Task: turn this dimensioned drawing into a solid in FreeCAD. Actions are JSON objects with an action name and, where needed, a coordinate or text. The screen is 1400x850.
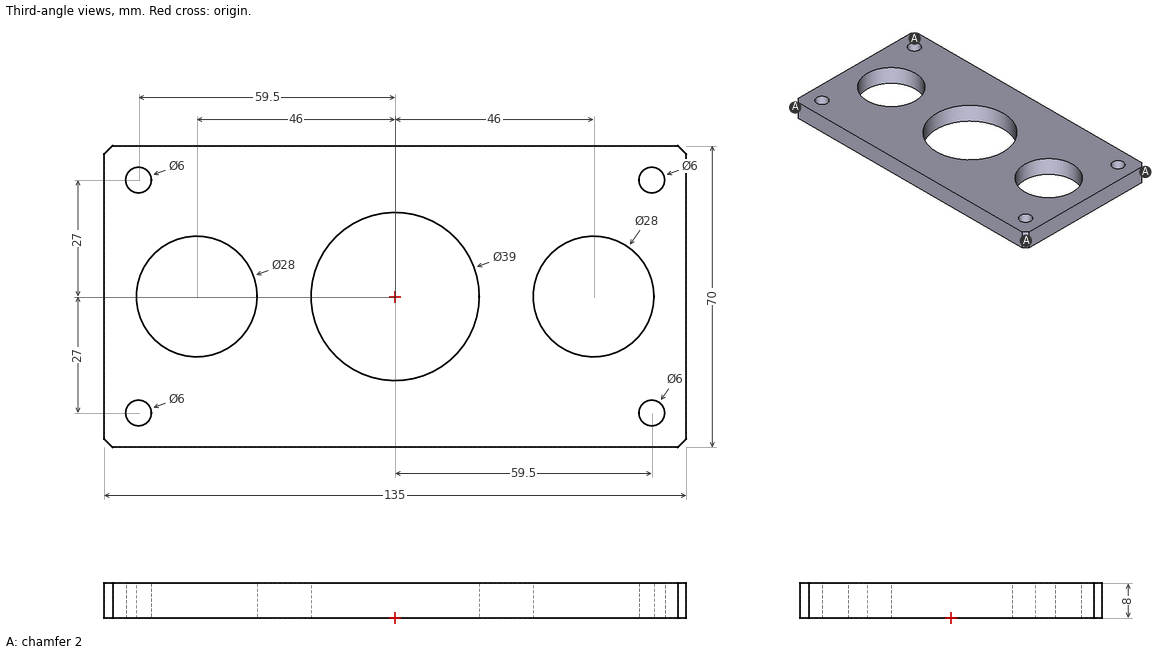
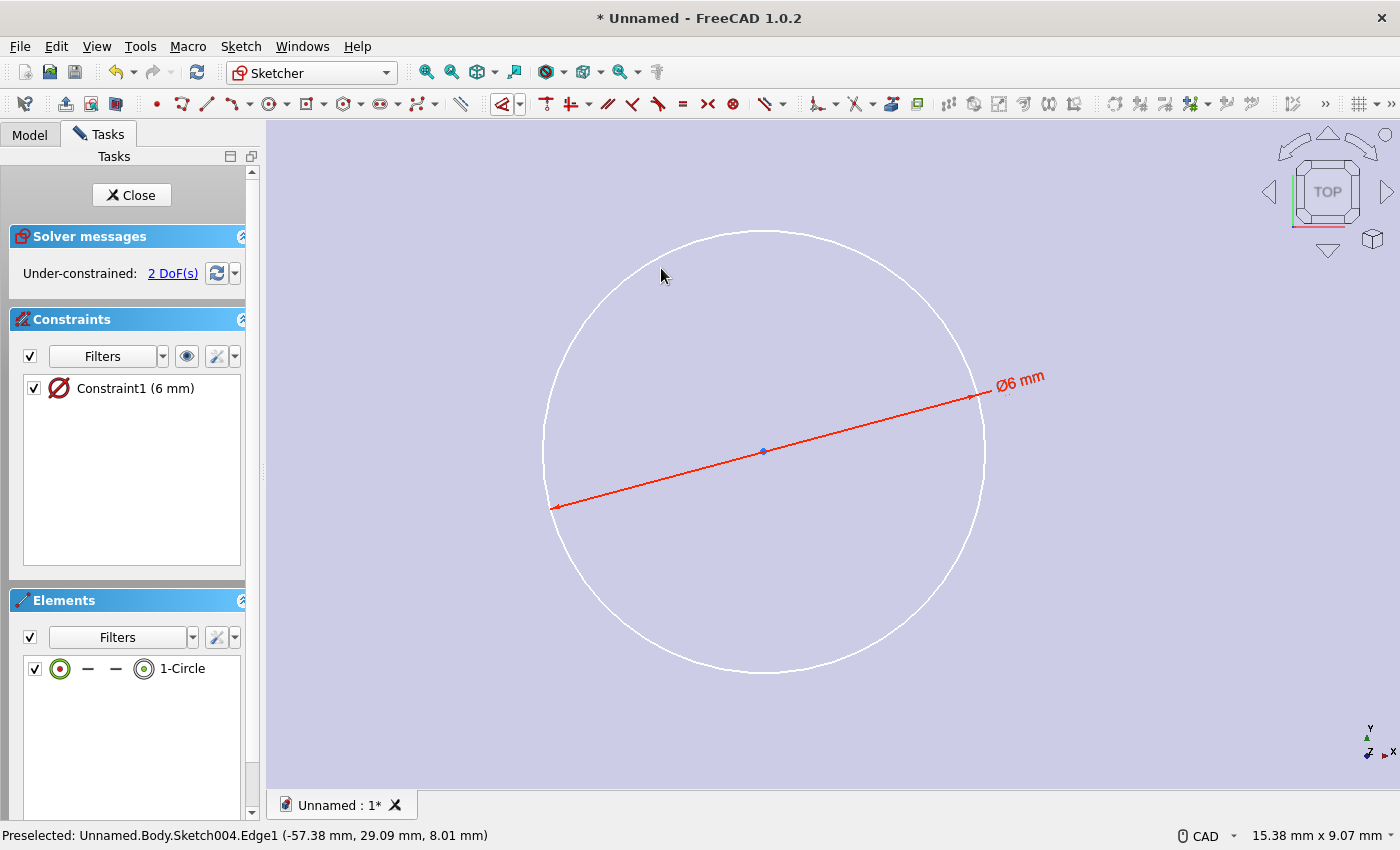
{"action": "left_click", "coordinate": [764, 452]}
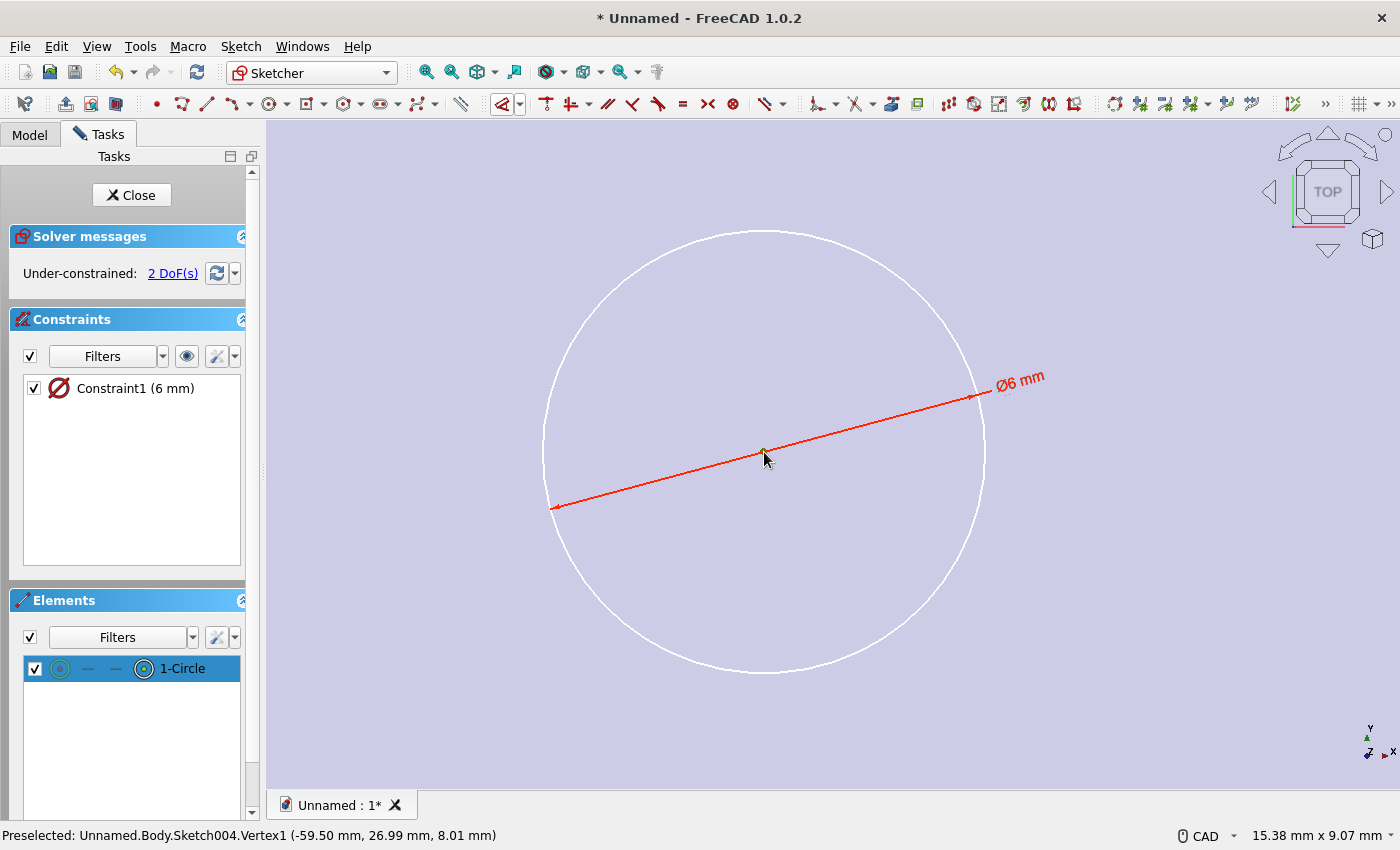
{"action": "key", "text": "i"}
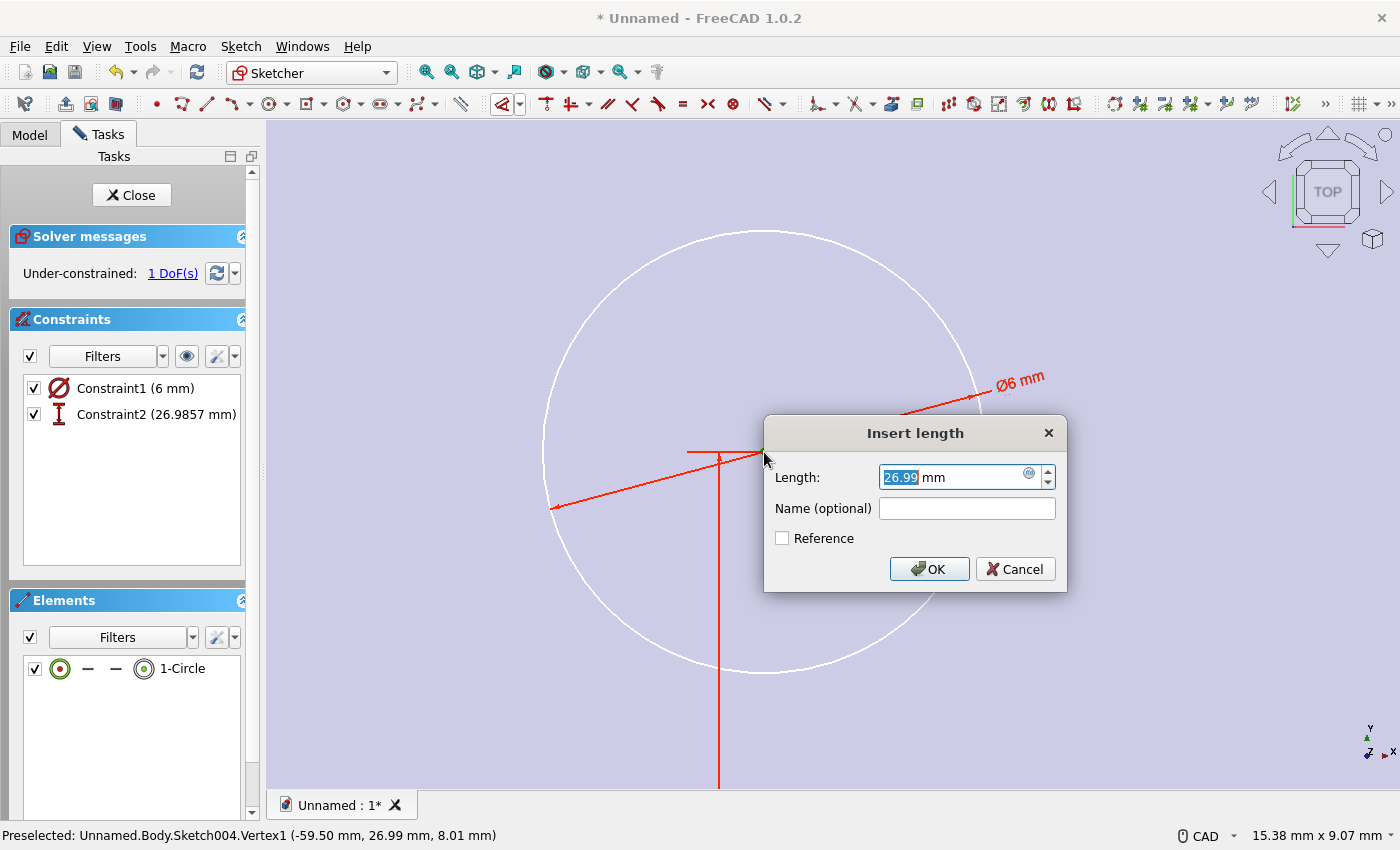
{"action": "type", "text": "27"}
{"action": "key", "text": "Return"}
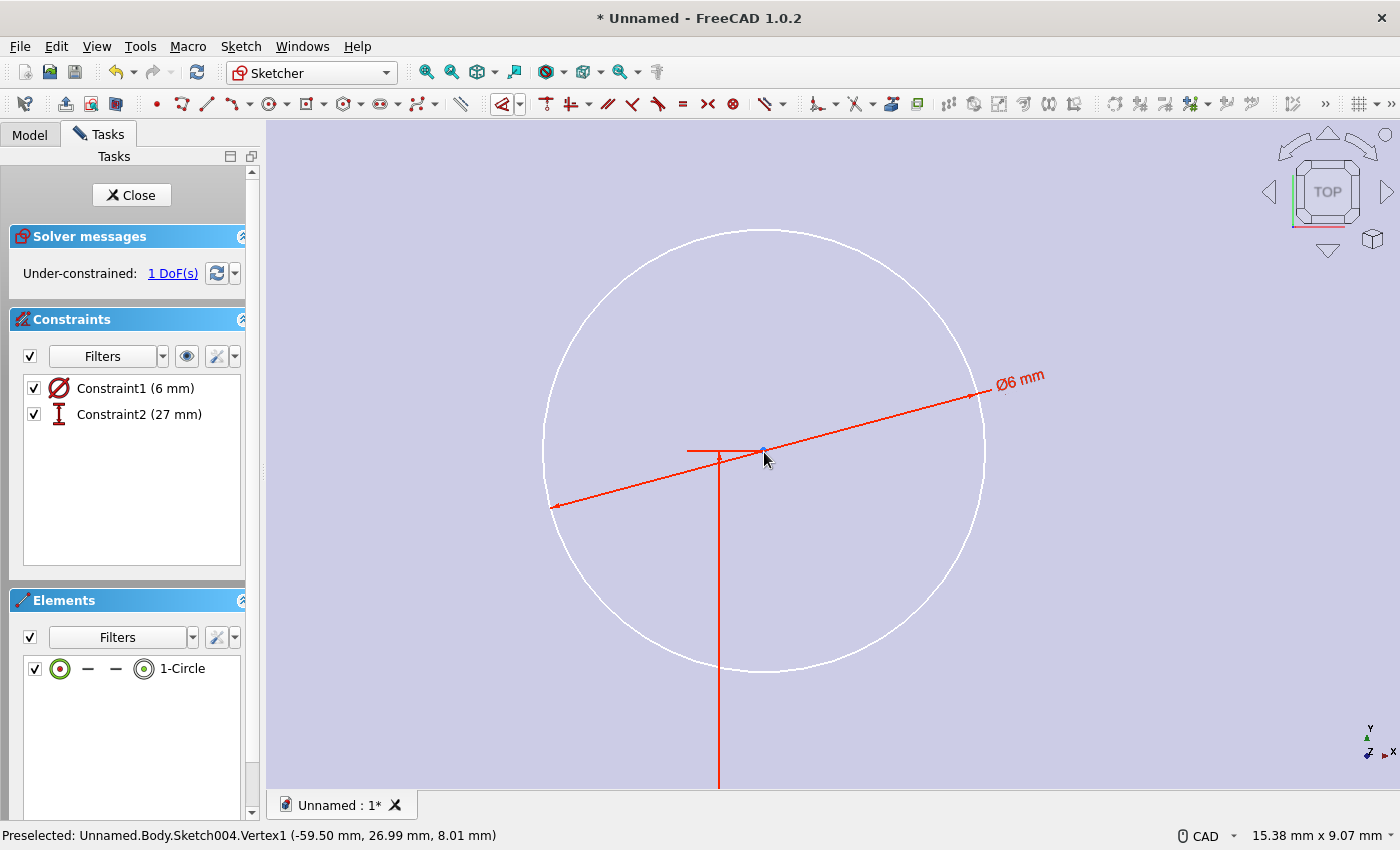
{"action": "left_click", "coordinate": [764, 451]}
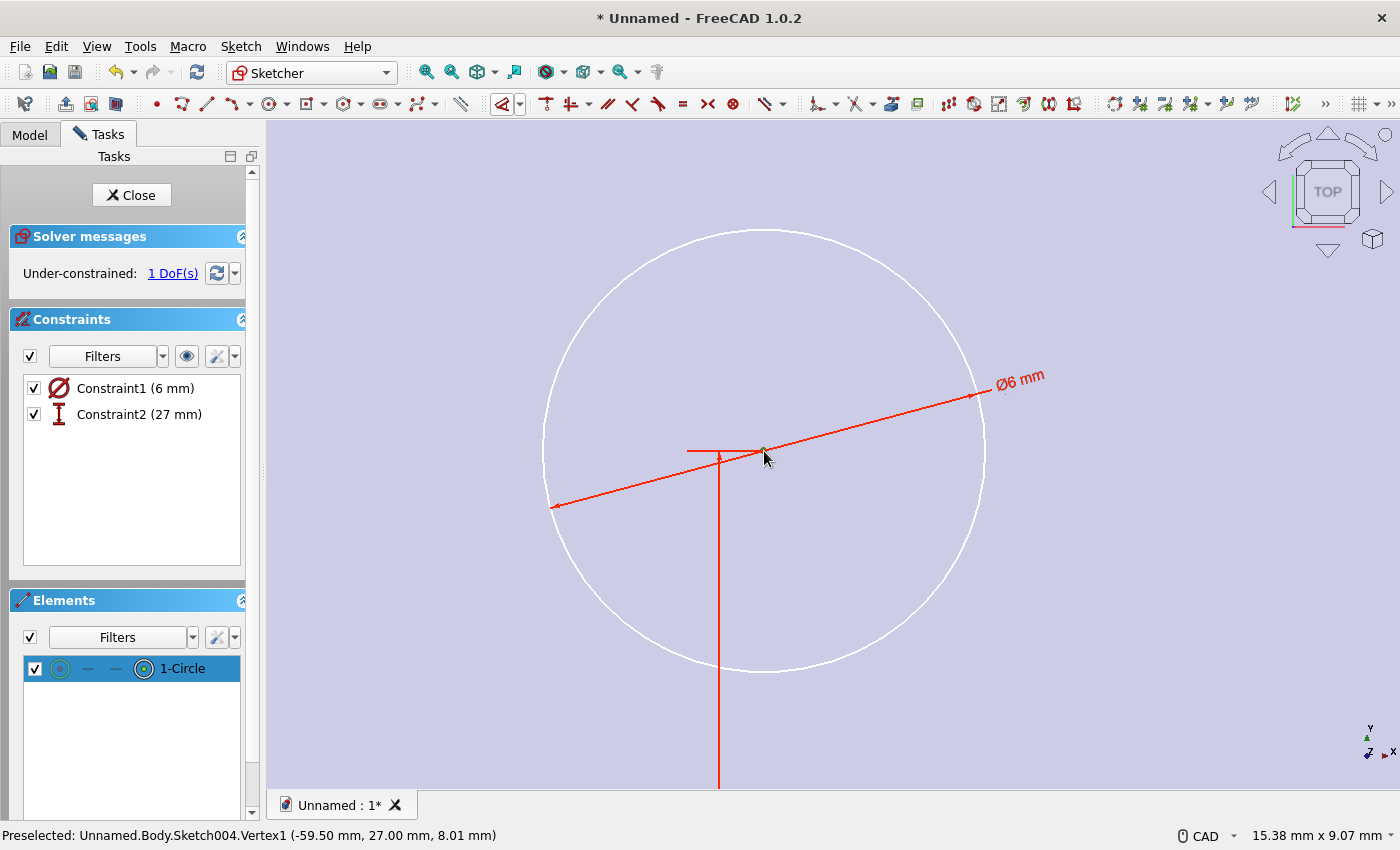
{"action": "key", "text": "l"}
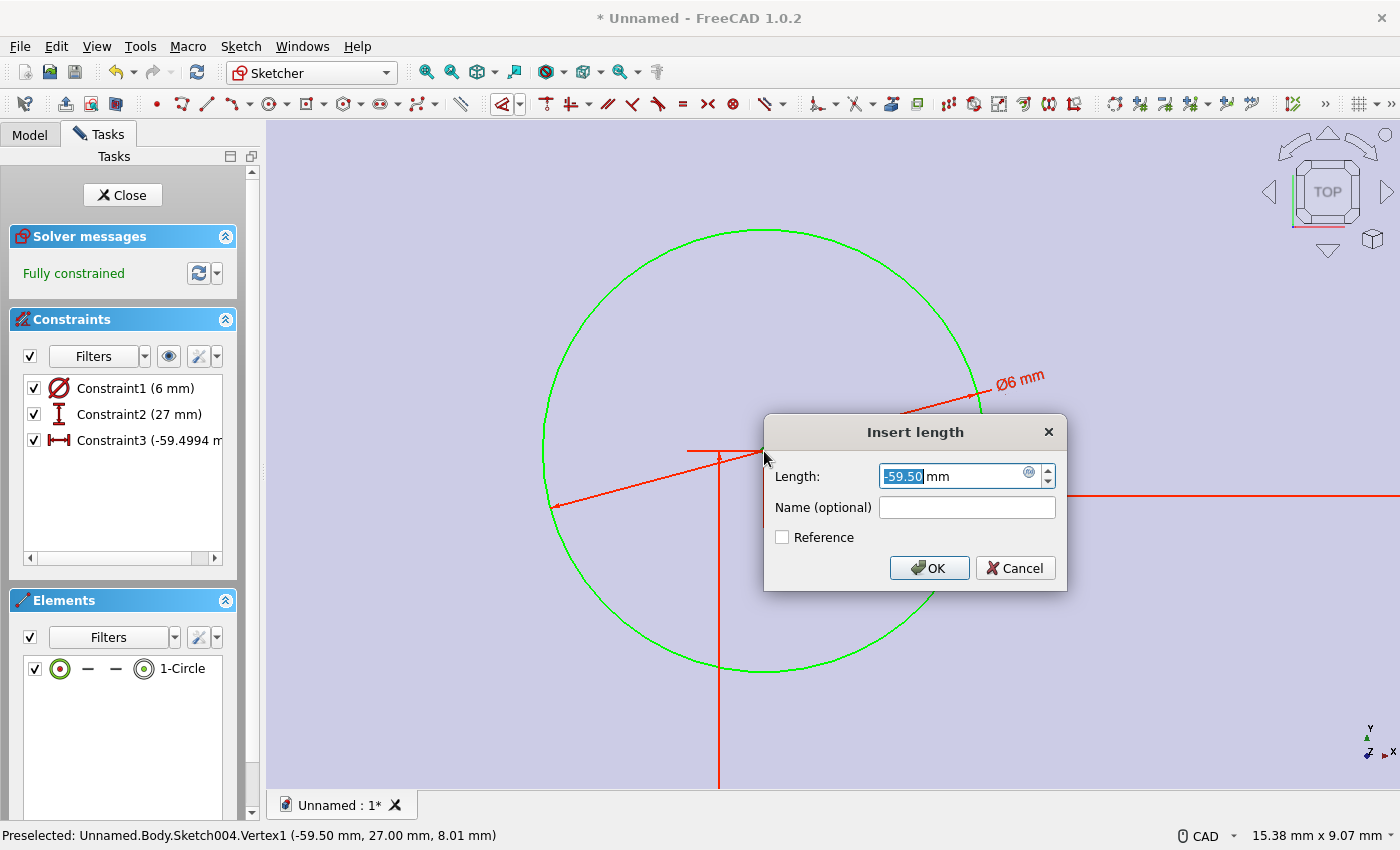
{"action": "type", "text": "-59.5"}
{"action": "key", "text": "Return"}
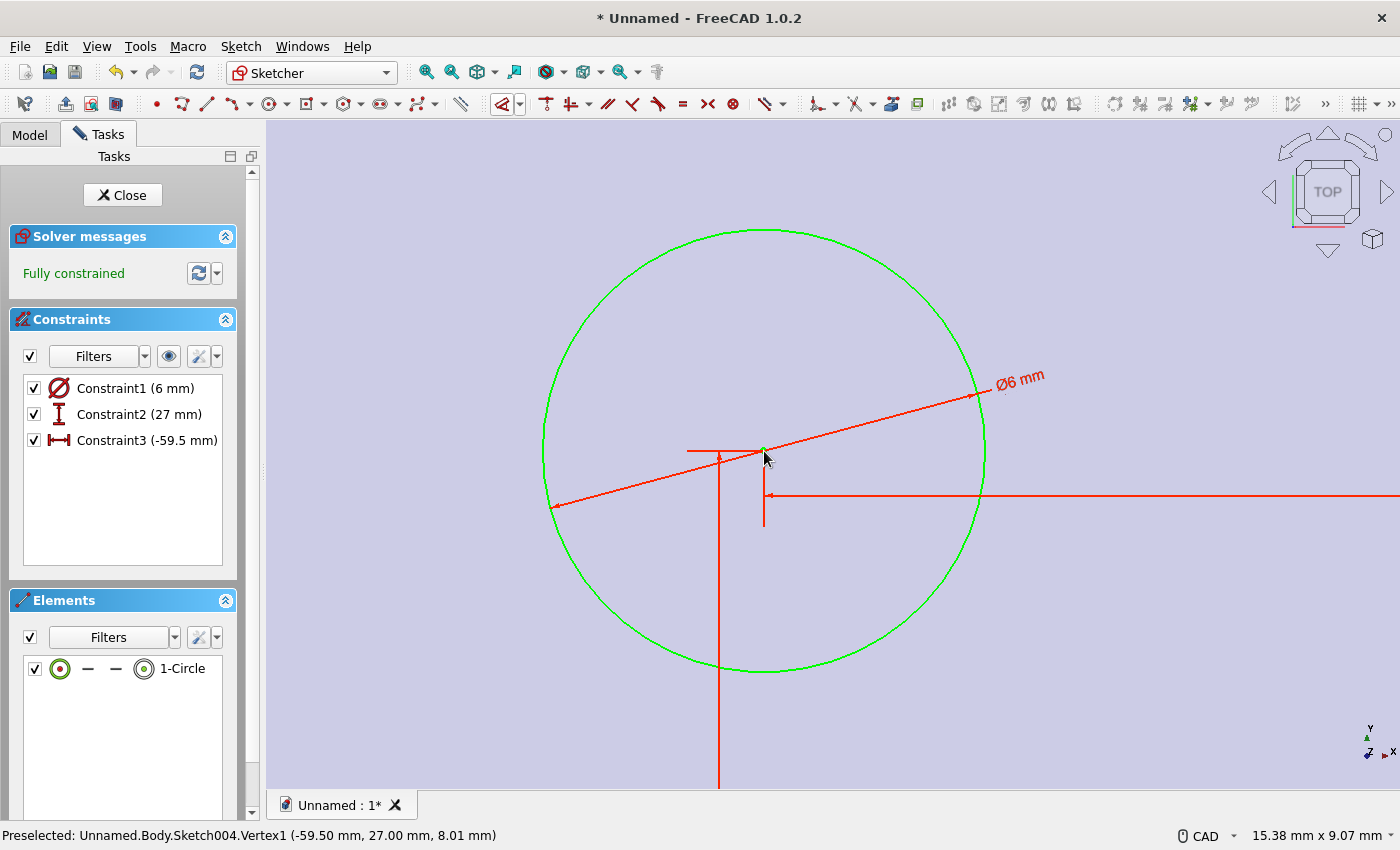
{"action": "left_click", "coordinate": [123, 195]}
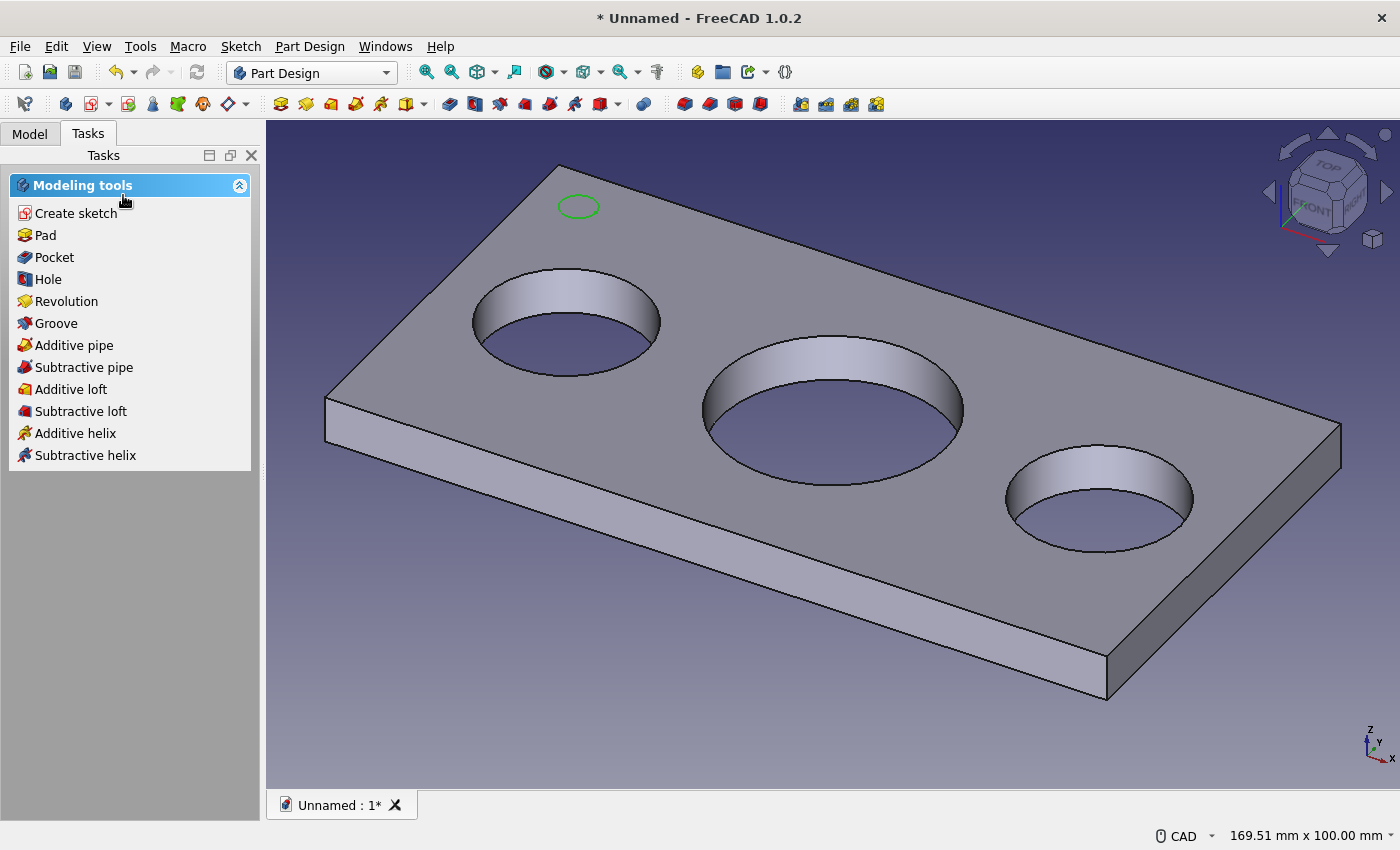
{"action": "left_click", "coordinate": [450, 104]}